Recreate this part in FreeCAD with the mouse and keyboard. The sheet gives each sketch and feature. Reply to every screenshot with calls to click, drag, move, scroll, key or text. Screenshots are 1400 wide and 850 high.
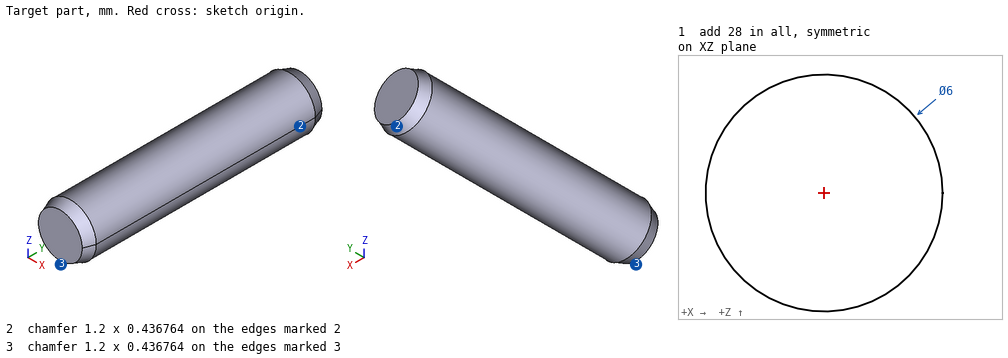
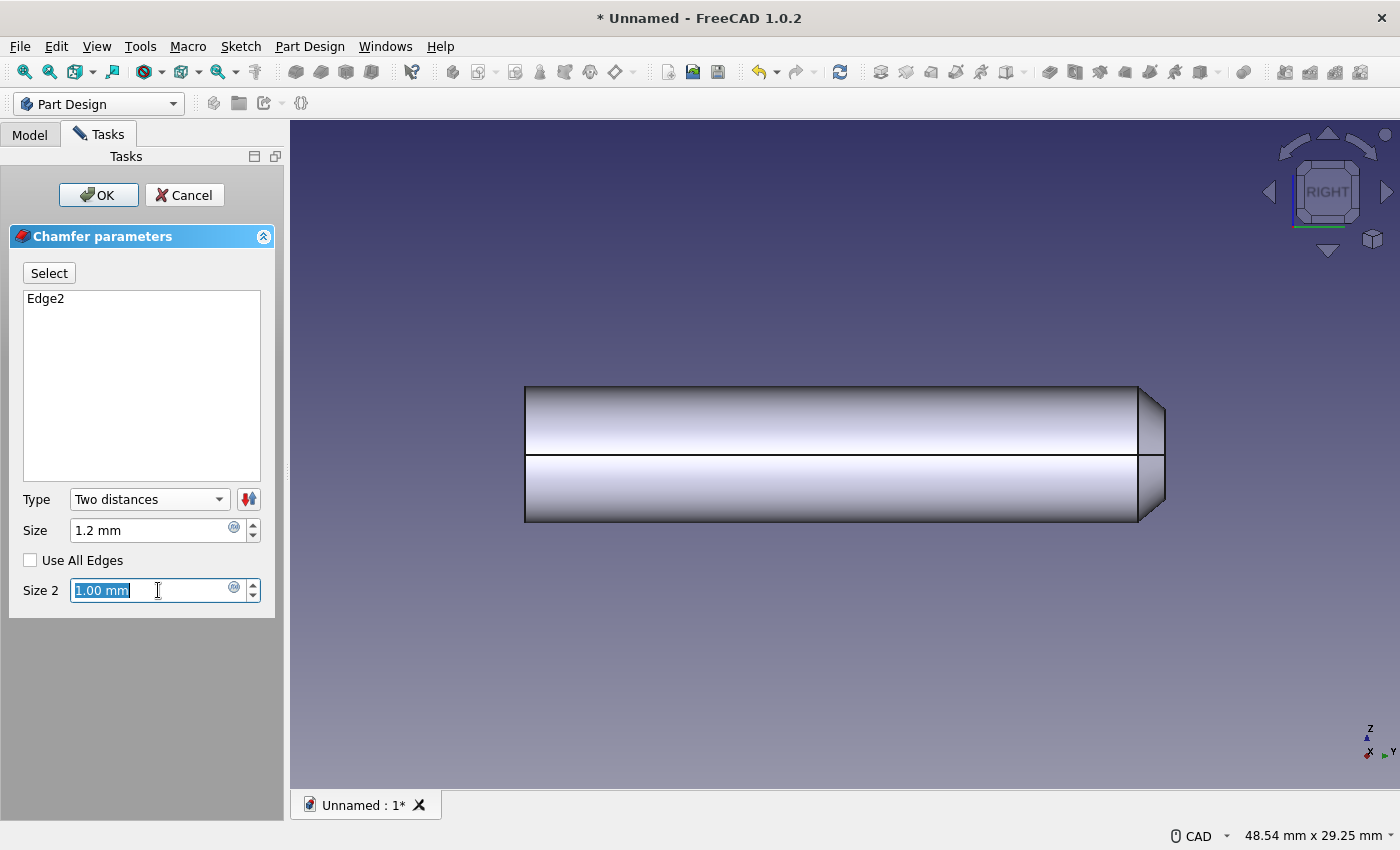
text(0.436764)
key(Tab)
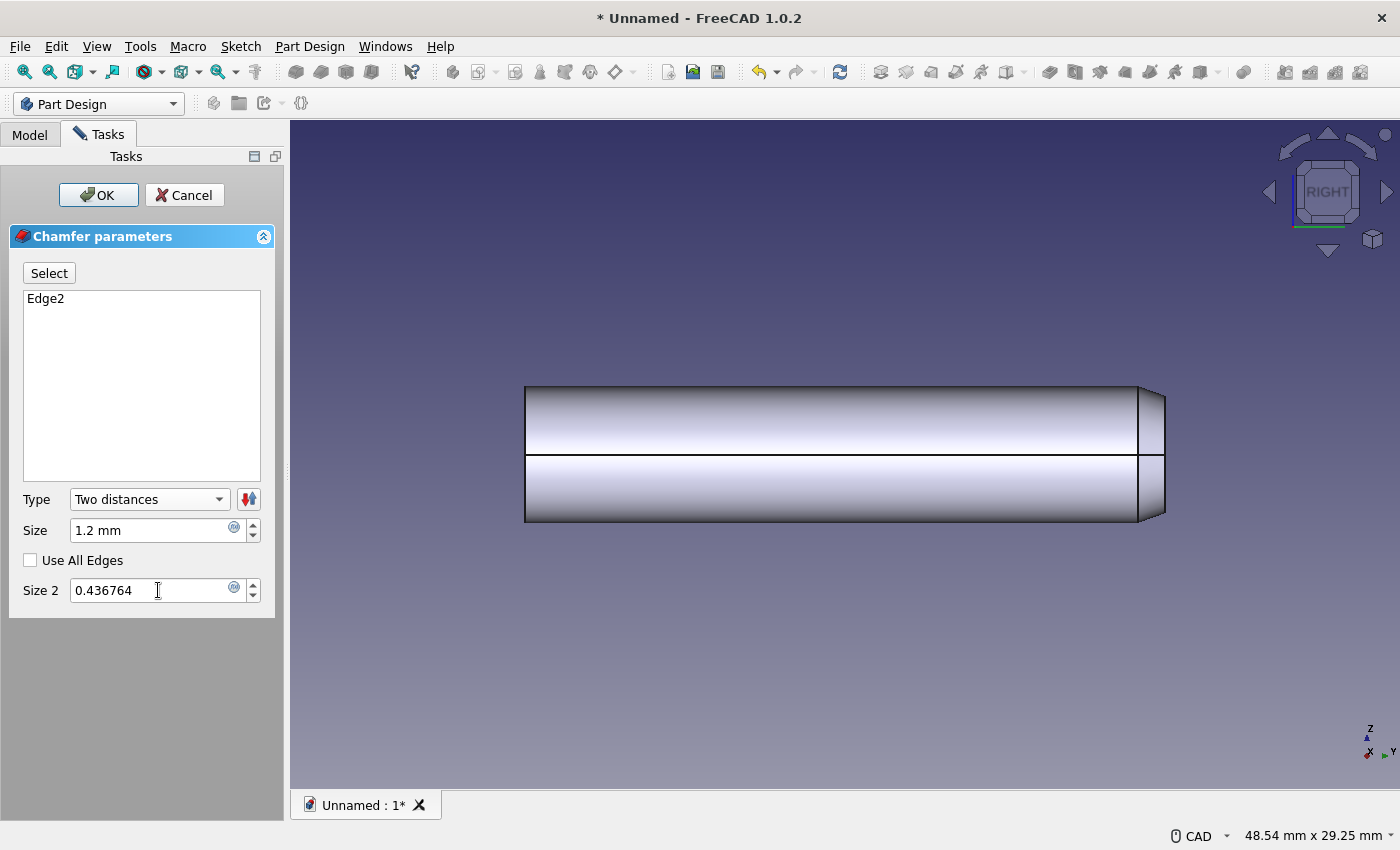
click(99, 195)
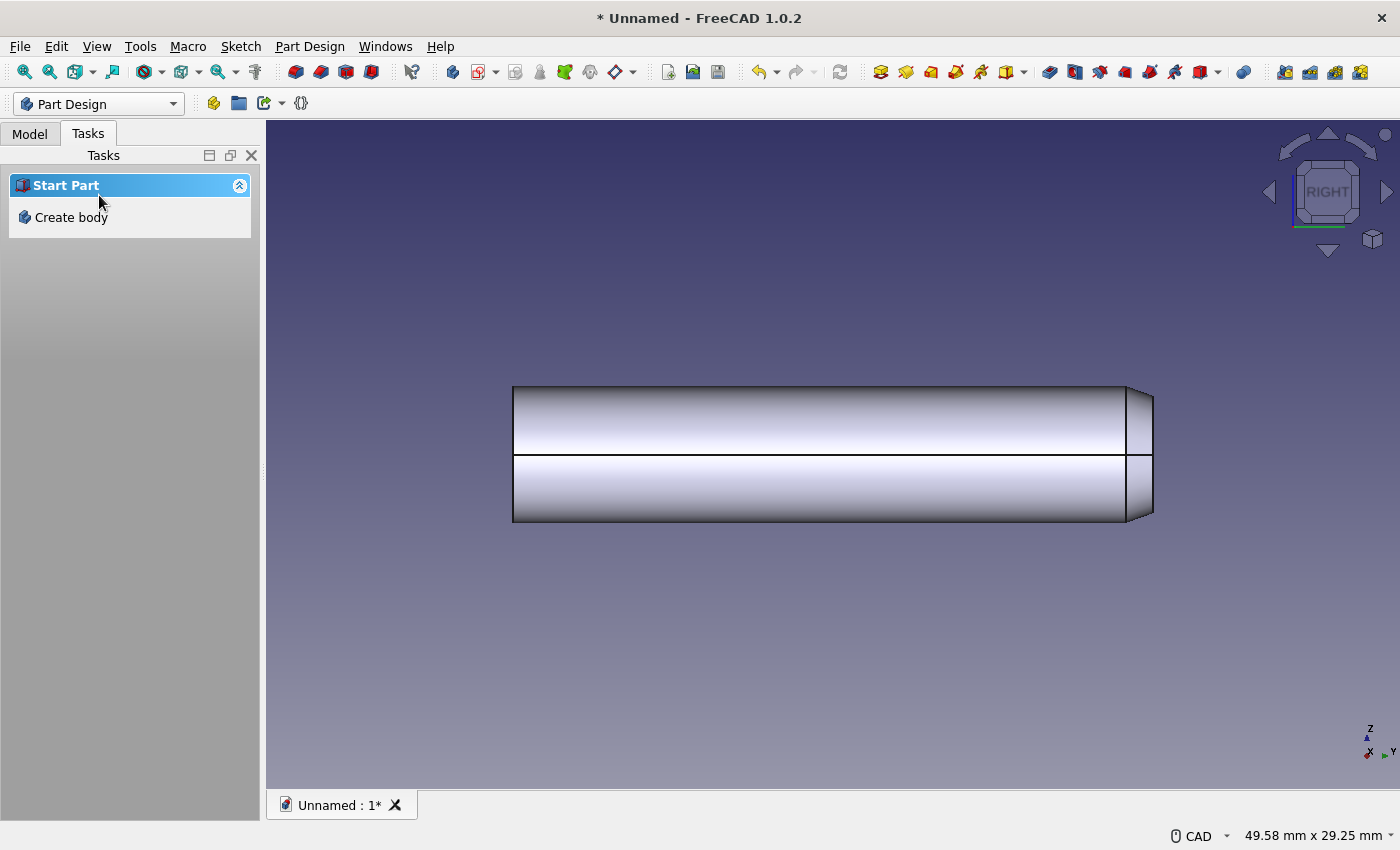
click(513, 413)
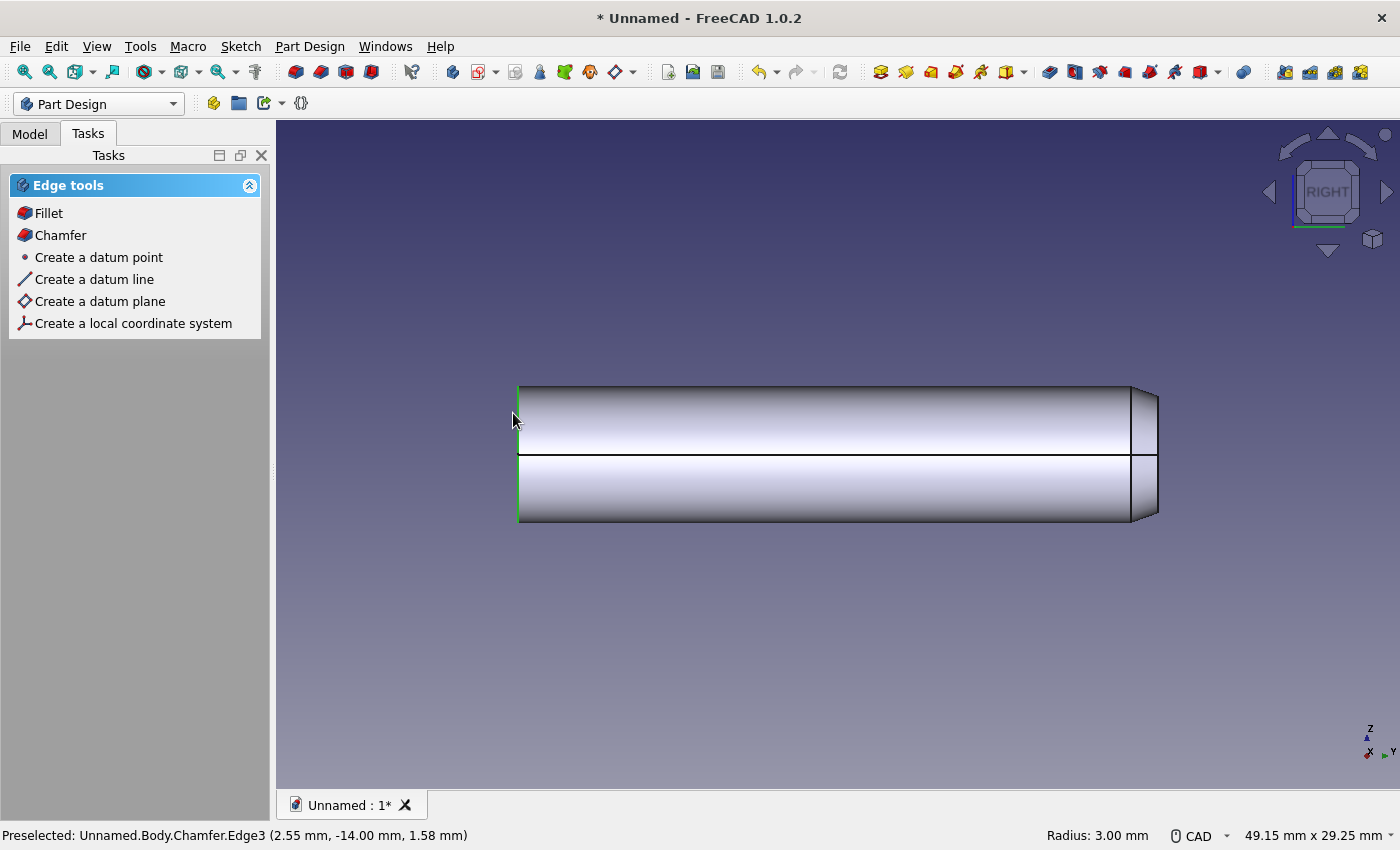
click(321, 72)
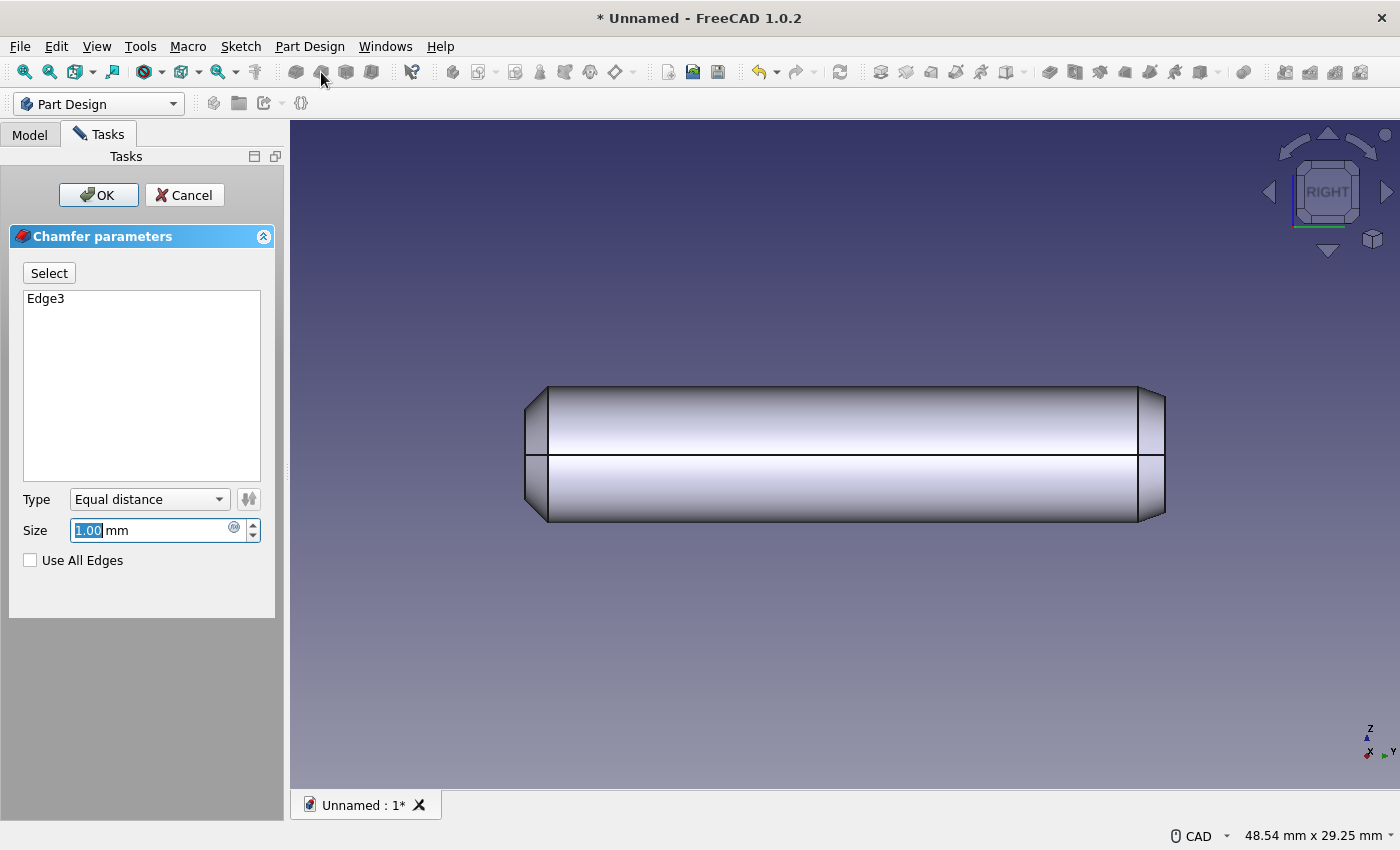
text(1.2)
key(Tab)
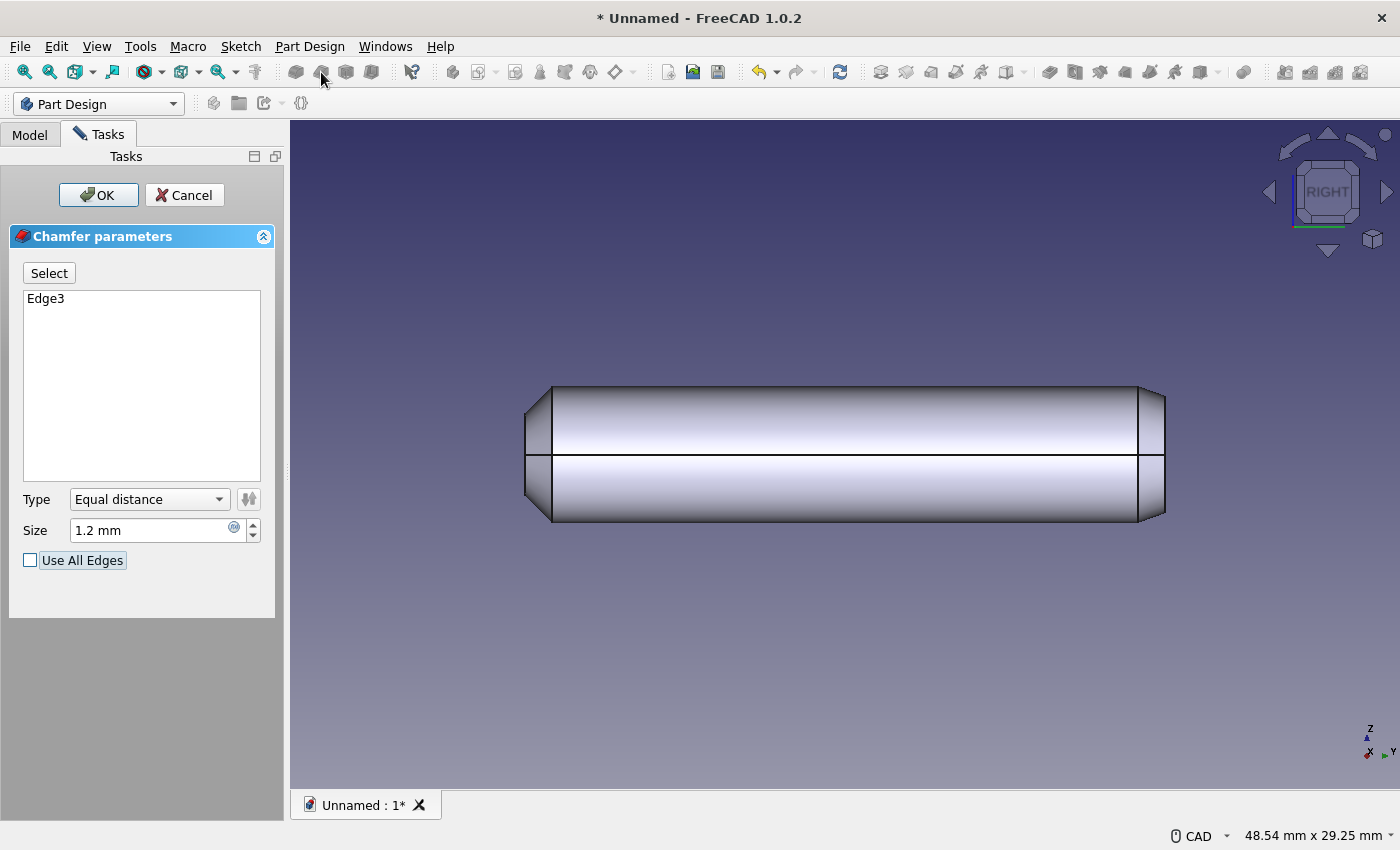
click(150, 500)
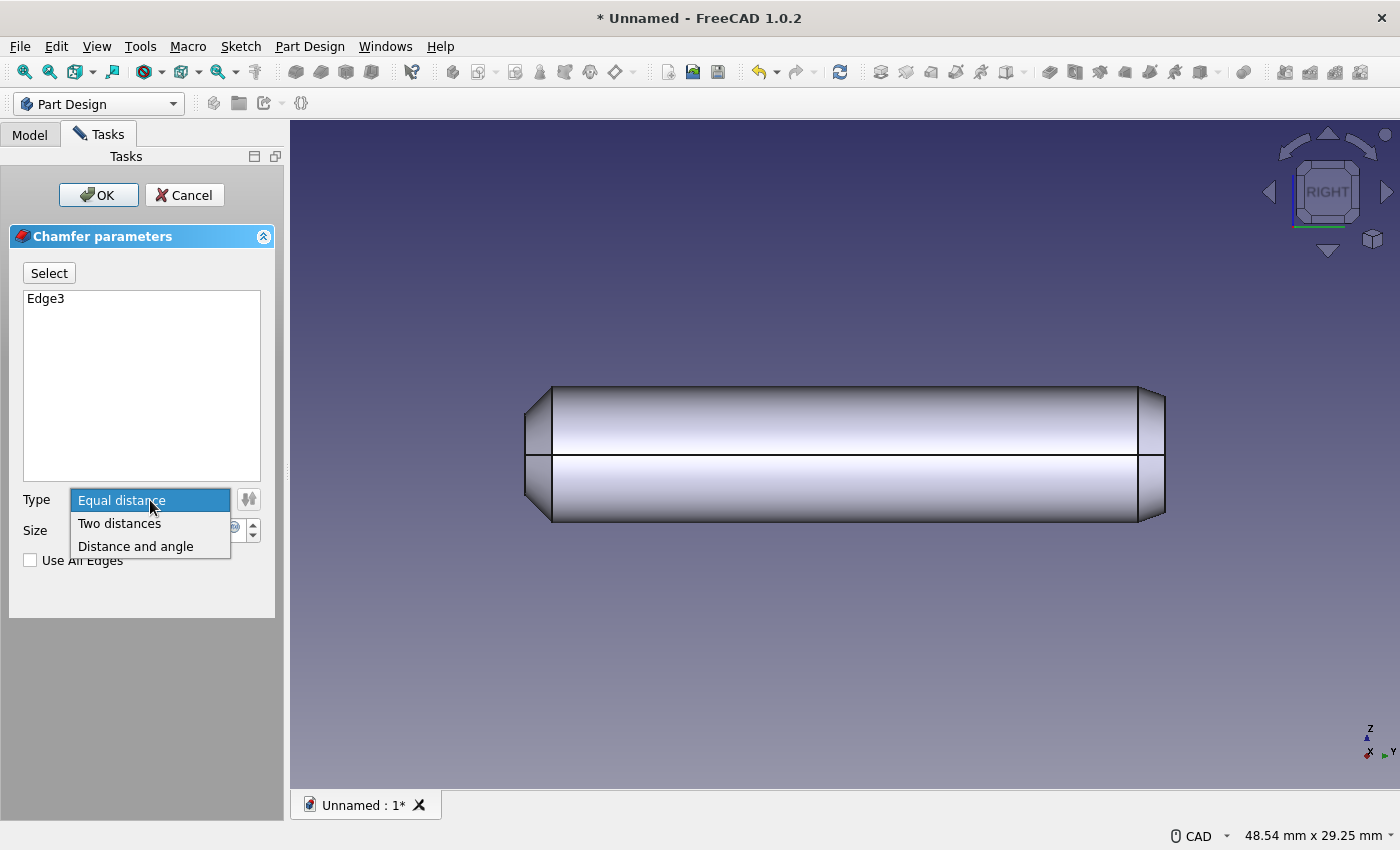
click(148, 524)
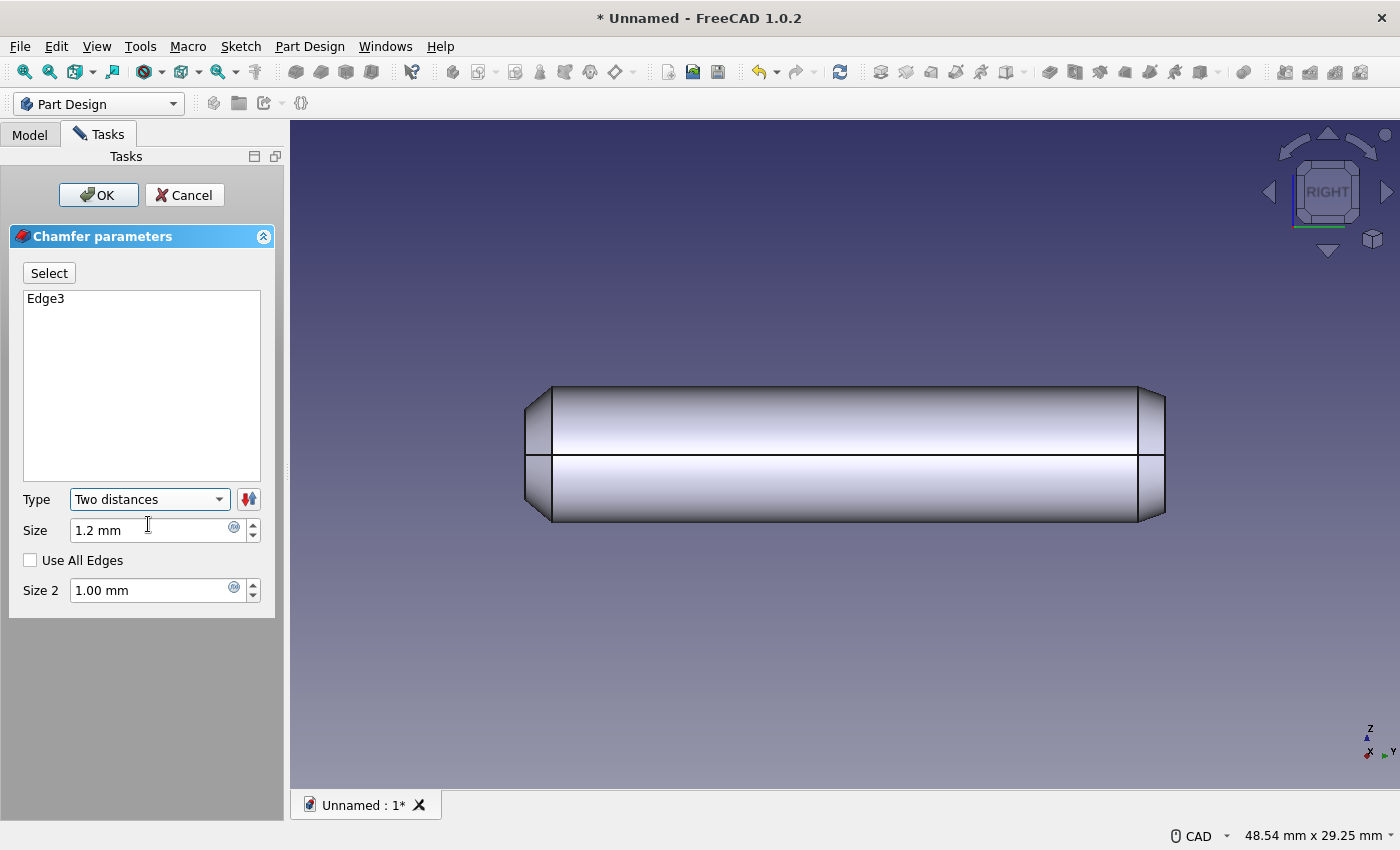
triple_click(158, 590)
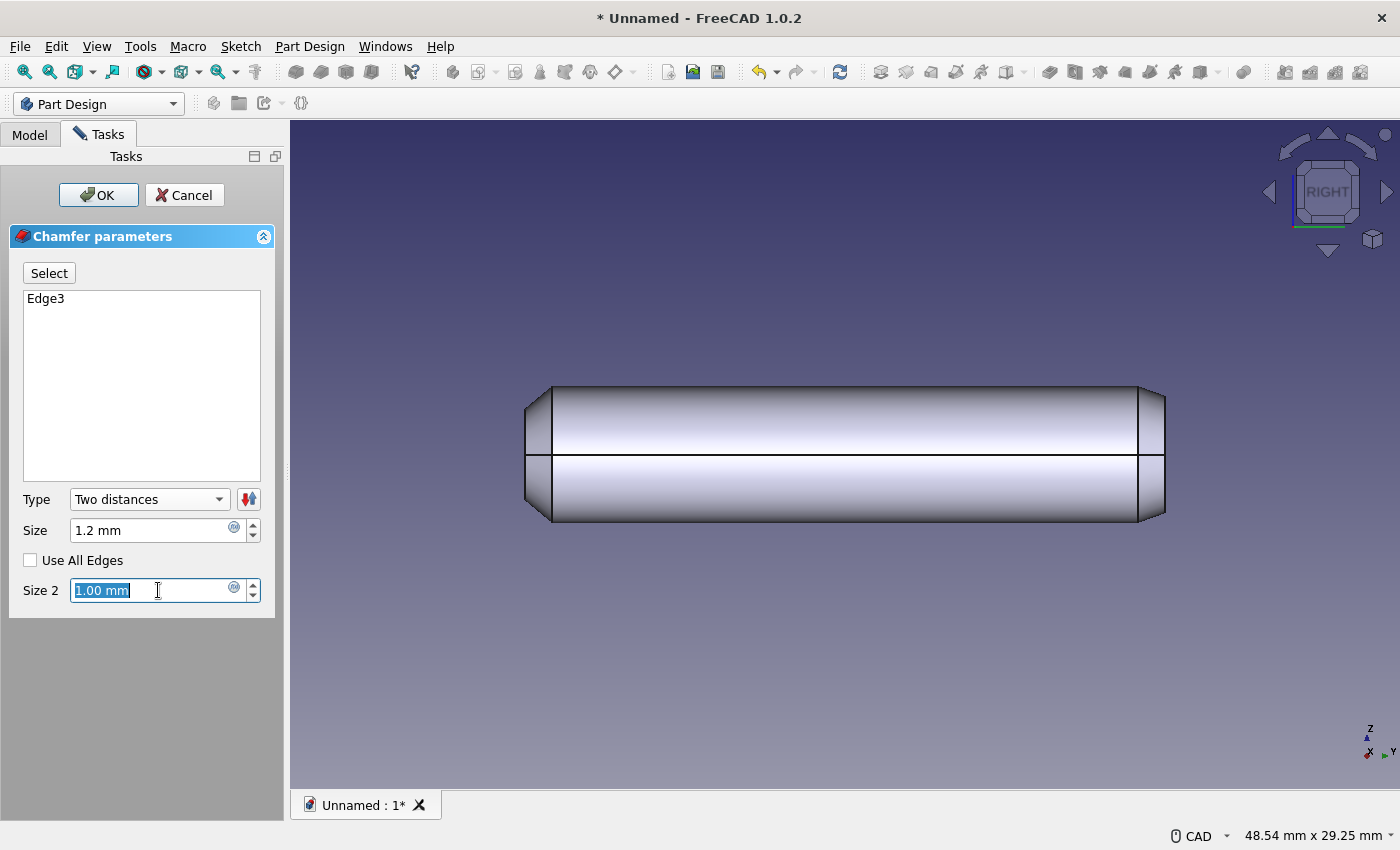
text(0.436764)
key(Tab)